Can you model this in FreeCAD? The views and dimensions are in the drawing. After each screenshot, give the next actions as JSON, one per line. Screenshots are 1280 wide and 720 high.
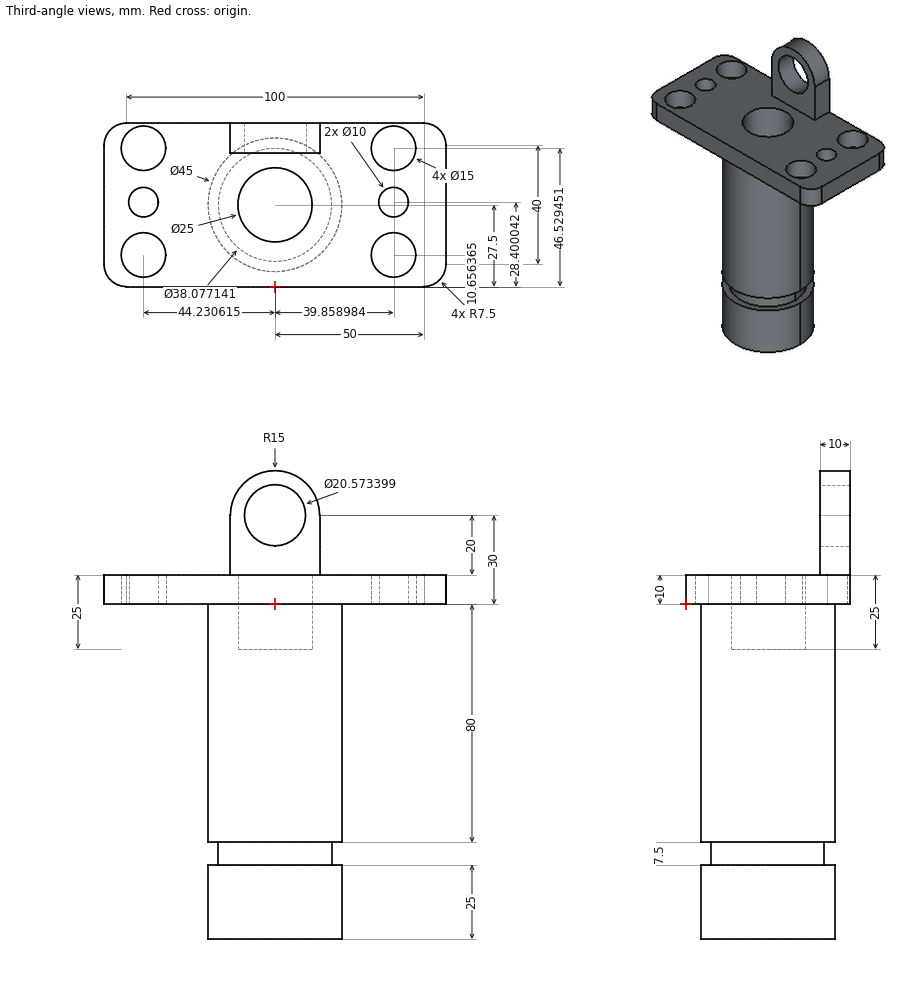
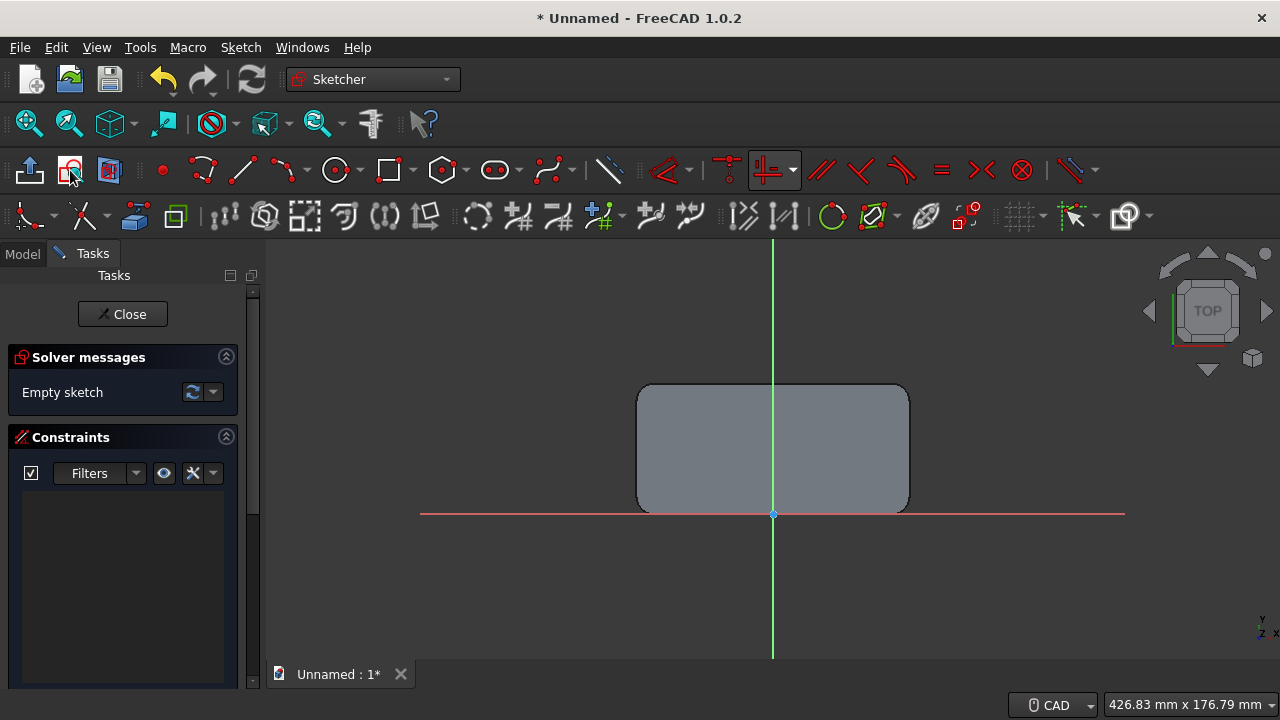
{"action": "scroll", "coordinate": [813, 477], "scroll_direction": "up", "scroll_amount": 5}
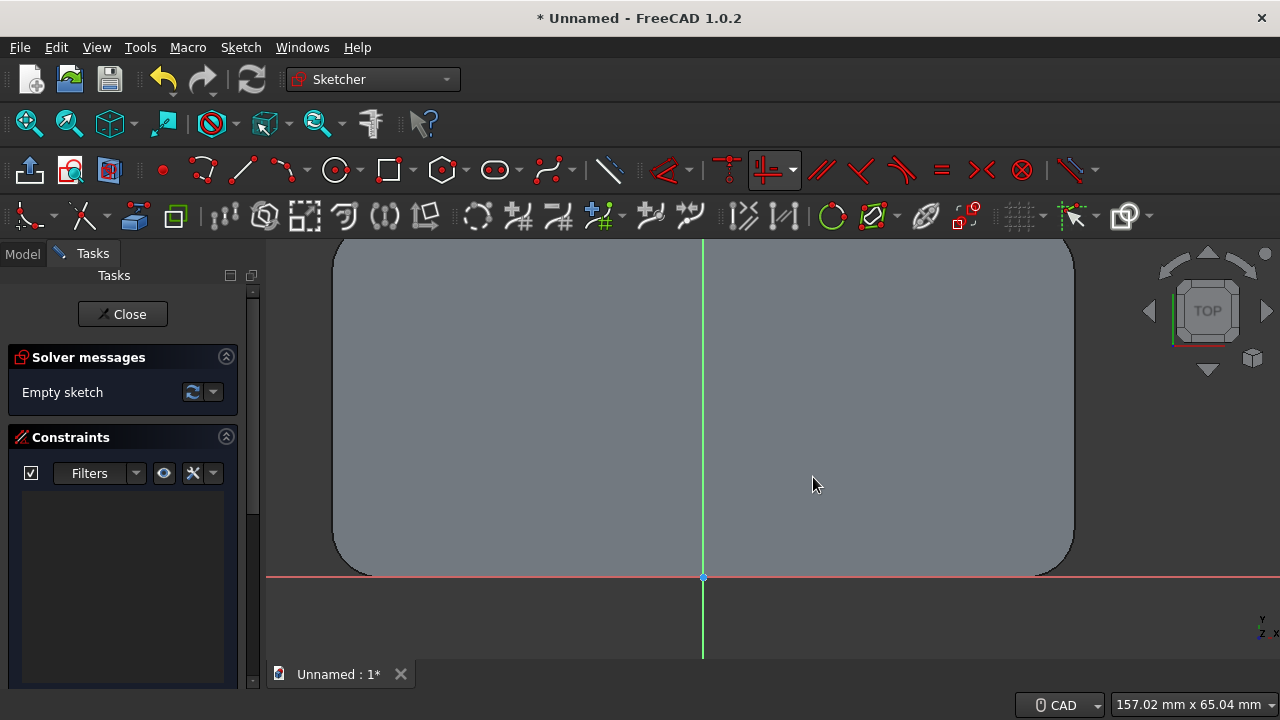
{"action": "left_click", "coordinate": [336, 170]}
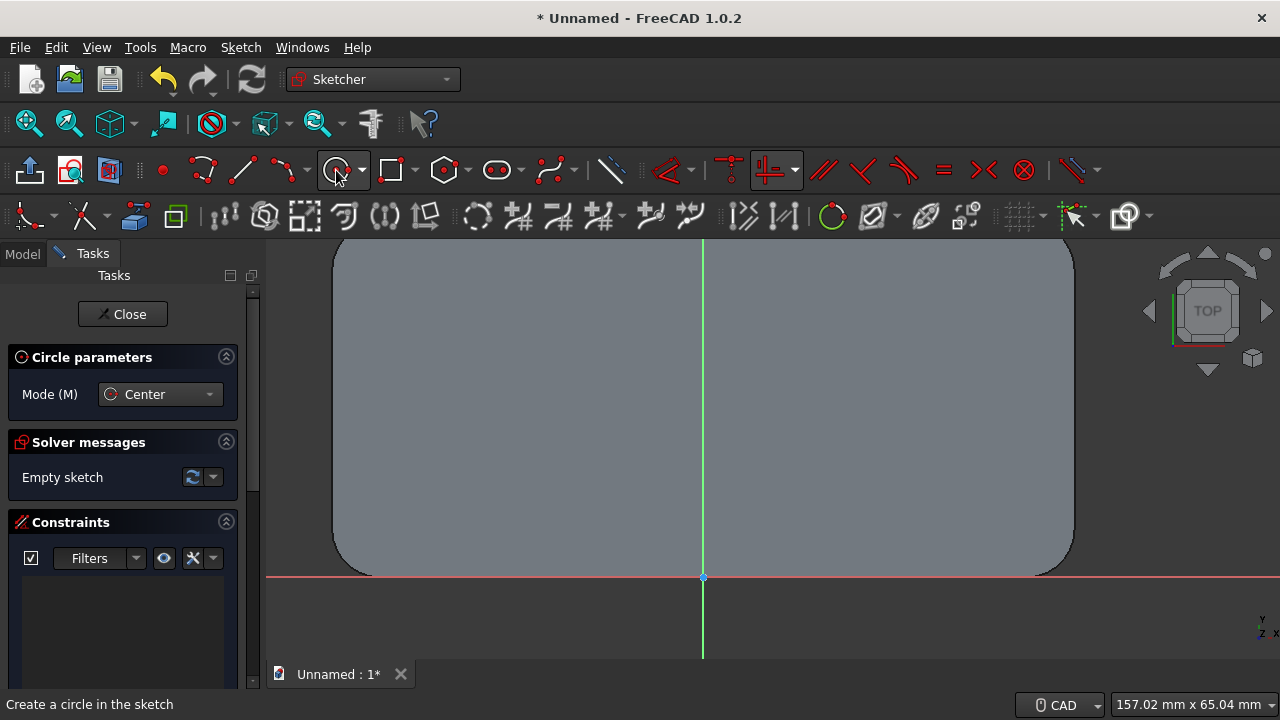
{"action": "left_click", "coordinate": [703, 400]}
{"action": "left_click", "coordinate": [760, 343]}
{"action": "key", "text": "Escape"}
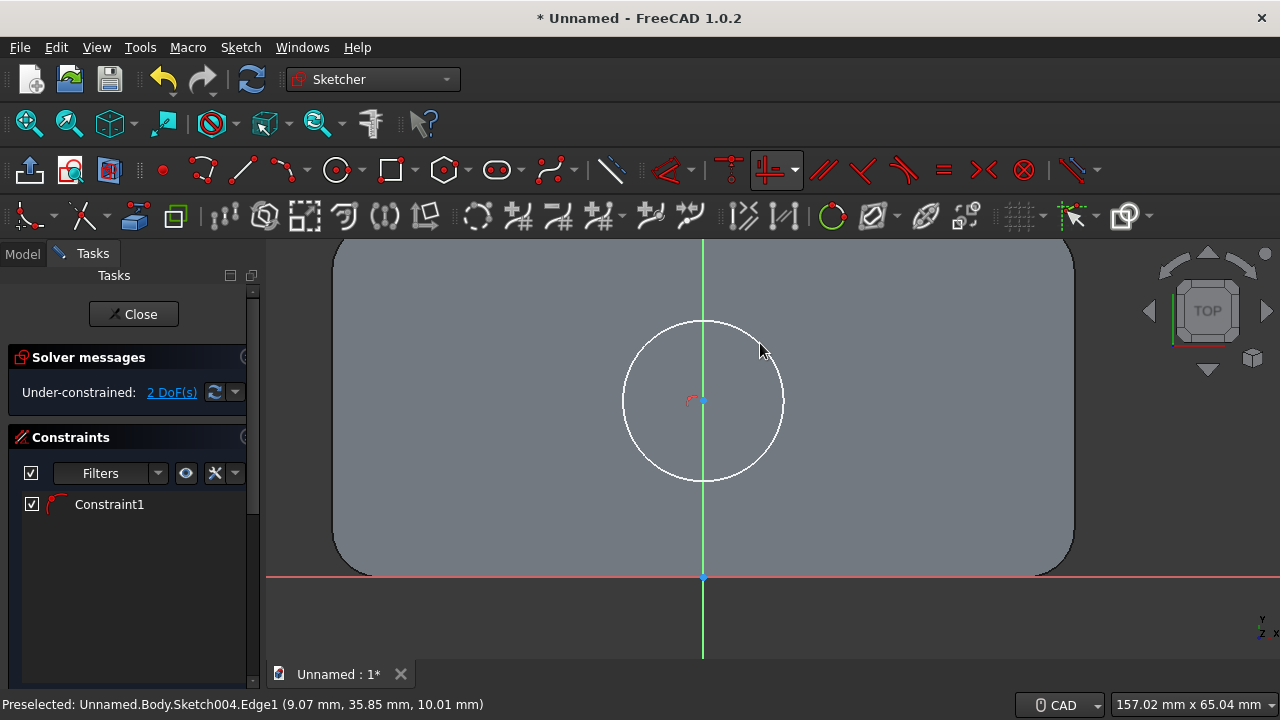
{"action": "left_click", "coordinate": [666, 170]}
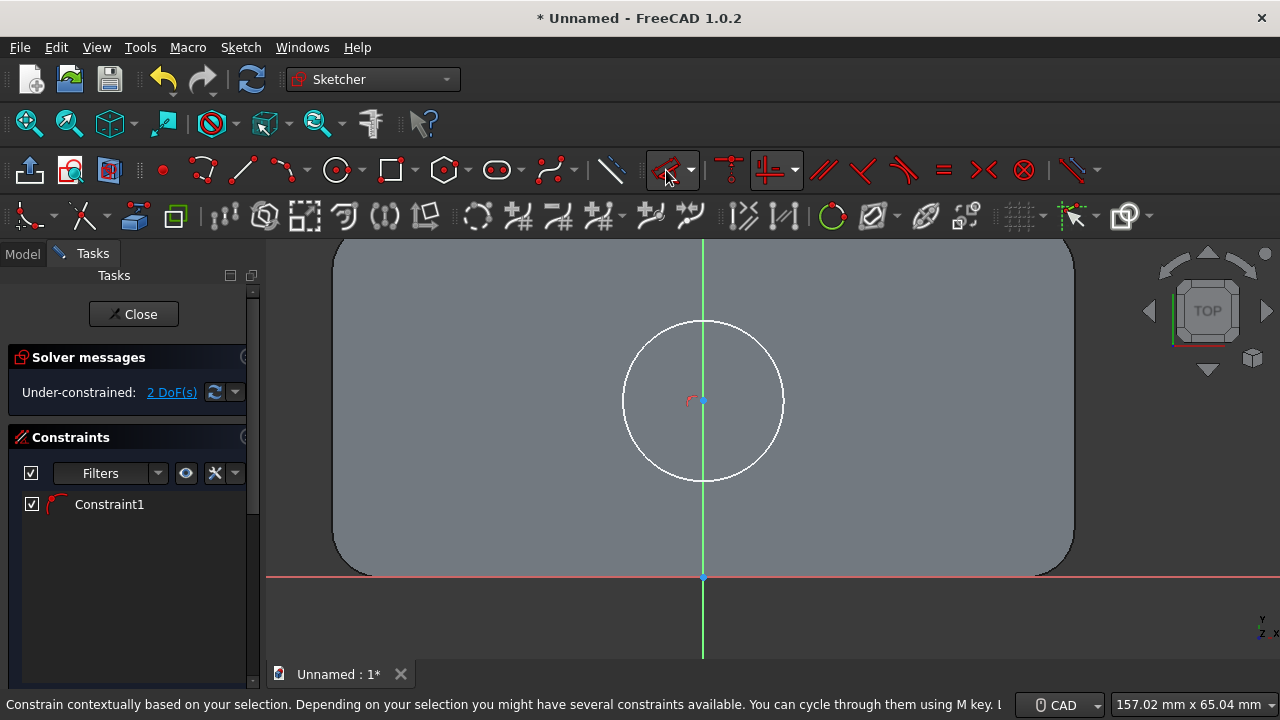
{"action": "left_click", "coordinate": [760, 344]}
{"action": "left_click", "coordinate": [783, 321]}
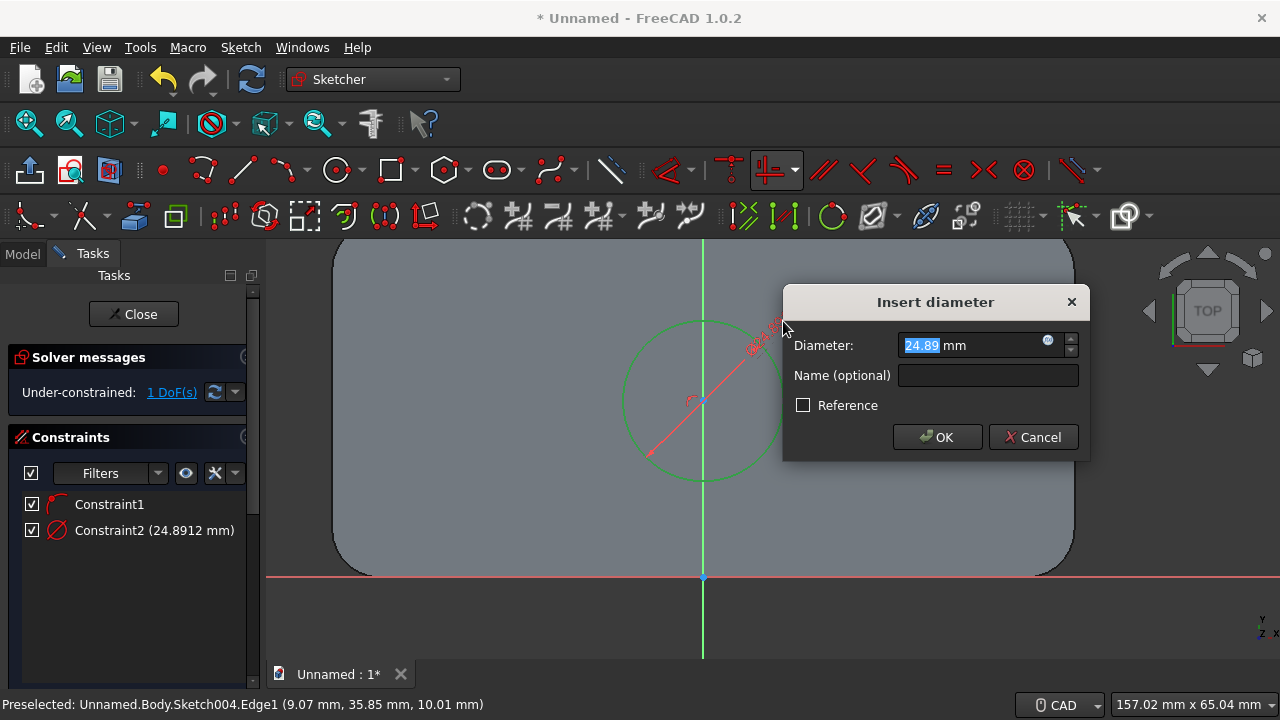
{"action": "type", "text": "25"}
{"action": "key", "text": "Return"}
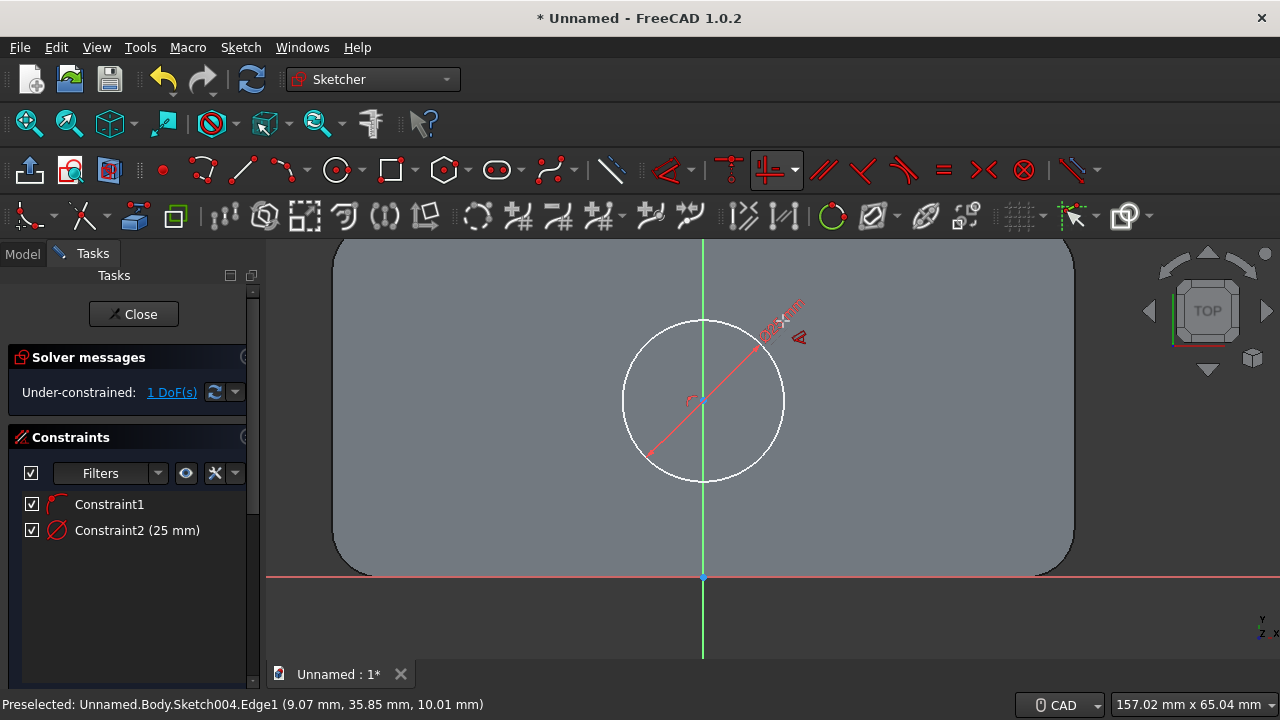
{"action": "left_click", "coordinate": [703, 401]}
{"action": "left_click", "coordinate": [737, 489]}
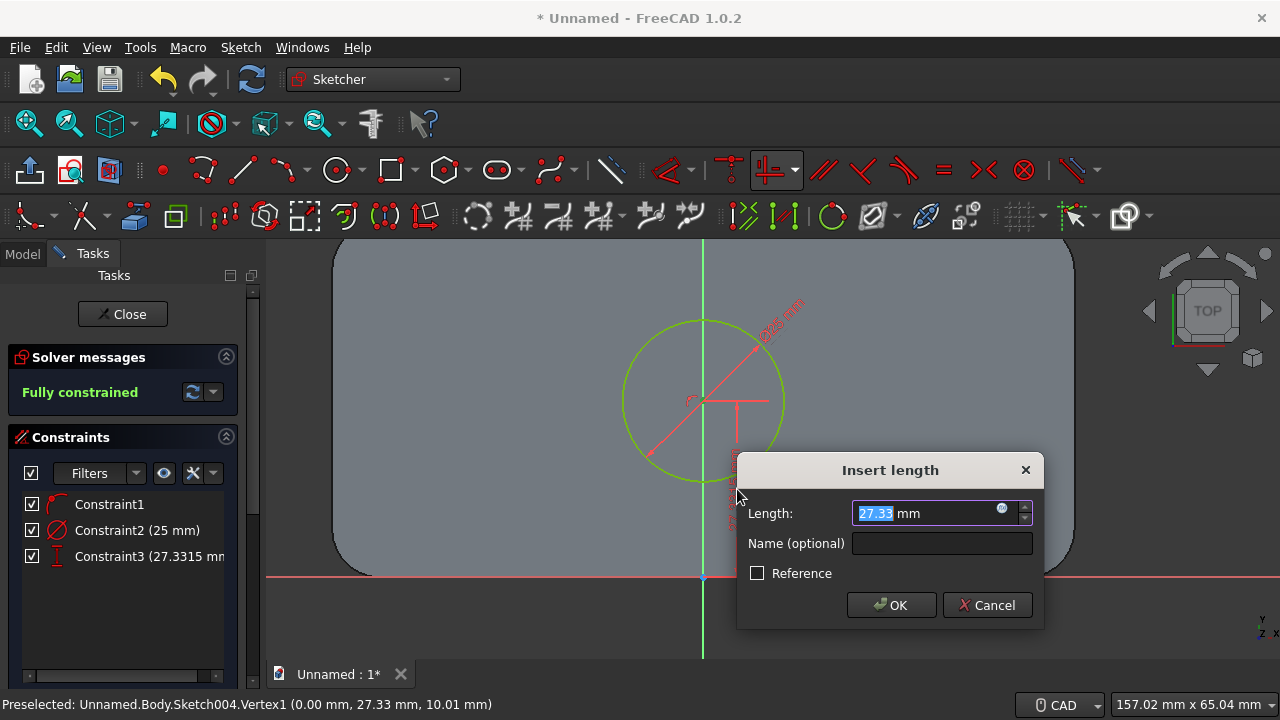
{"action": "type", "text": "27.5"}
{"action": "key", "text": "Return"}
{"action": "key", "text": "Escape"}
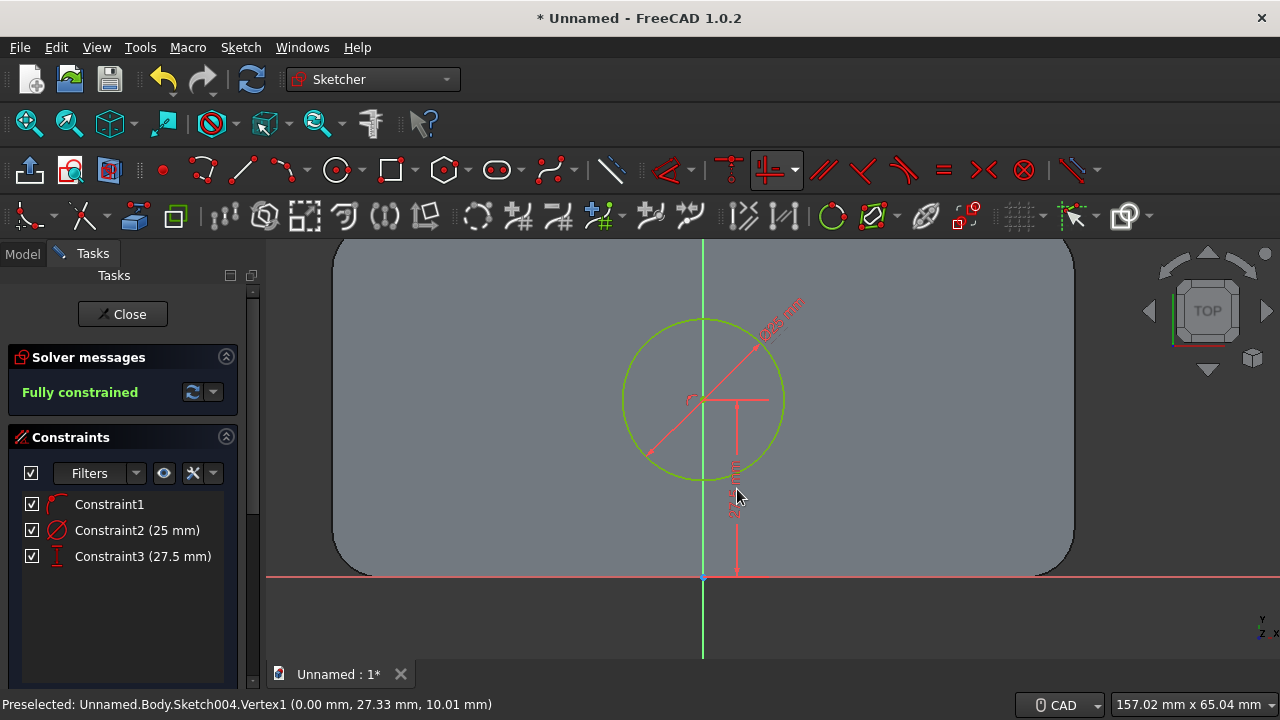
{"action": "left_click", "coordinate": [123, 314]}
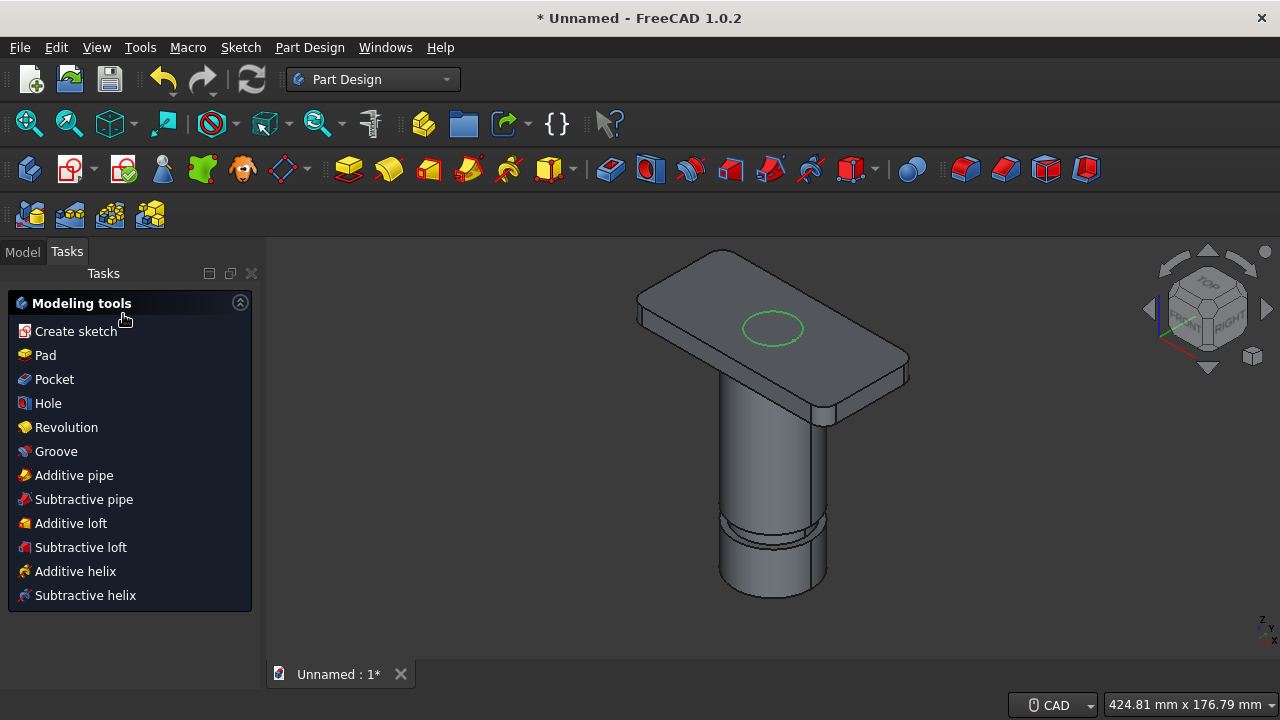
{"action": "left_click", "coordinate": [612, 170]}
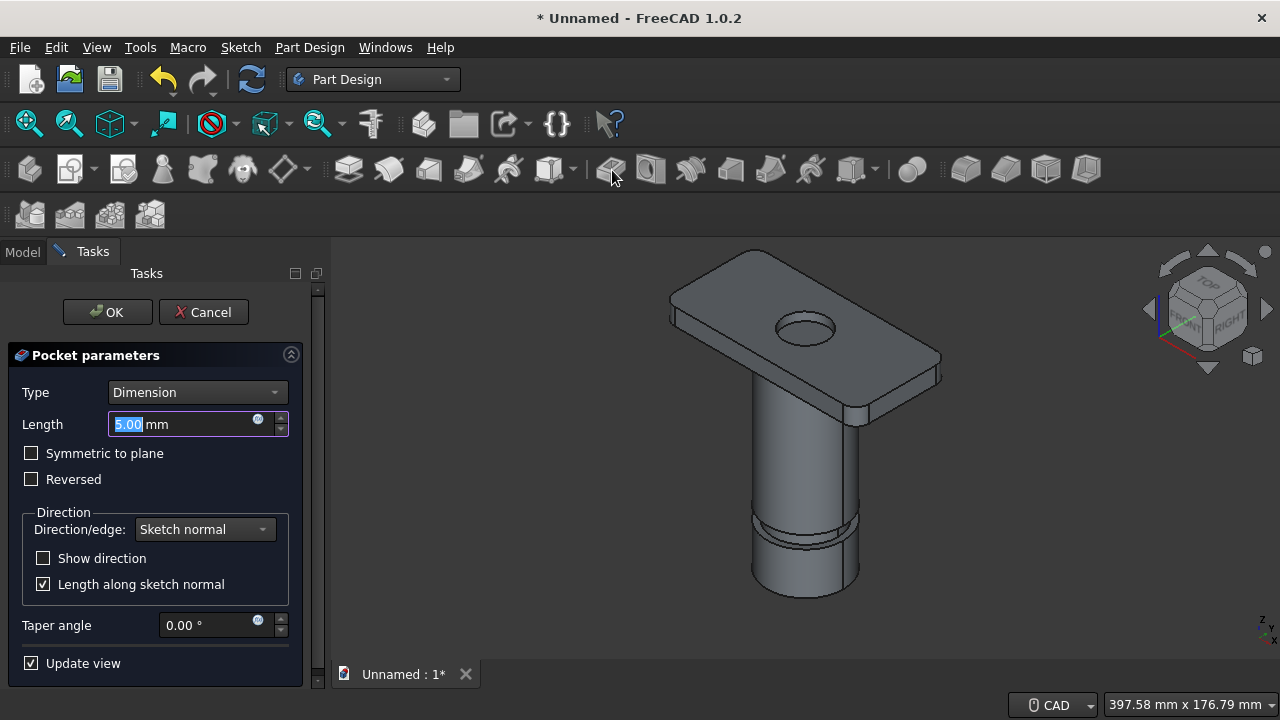
{"action": "type", "text": "25"}
{"action": "key", "text": "Tab"}